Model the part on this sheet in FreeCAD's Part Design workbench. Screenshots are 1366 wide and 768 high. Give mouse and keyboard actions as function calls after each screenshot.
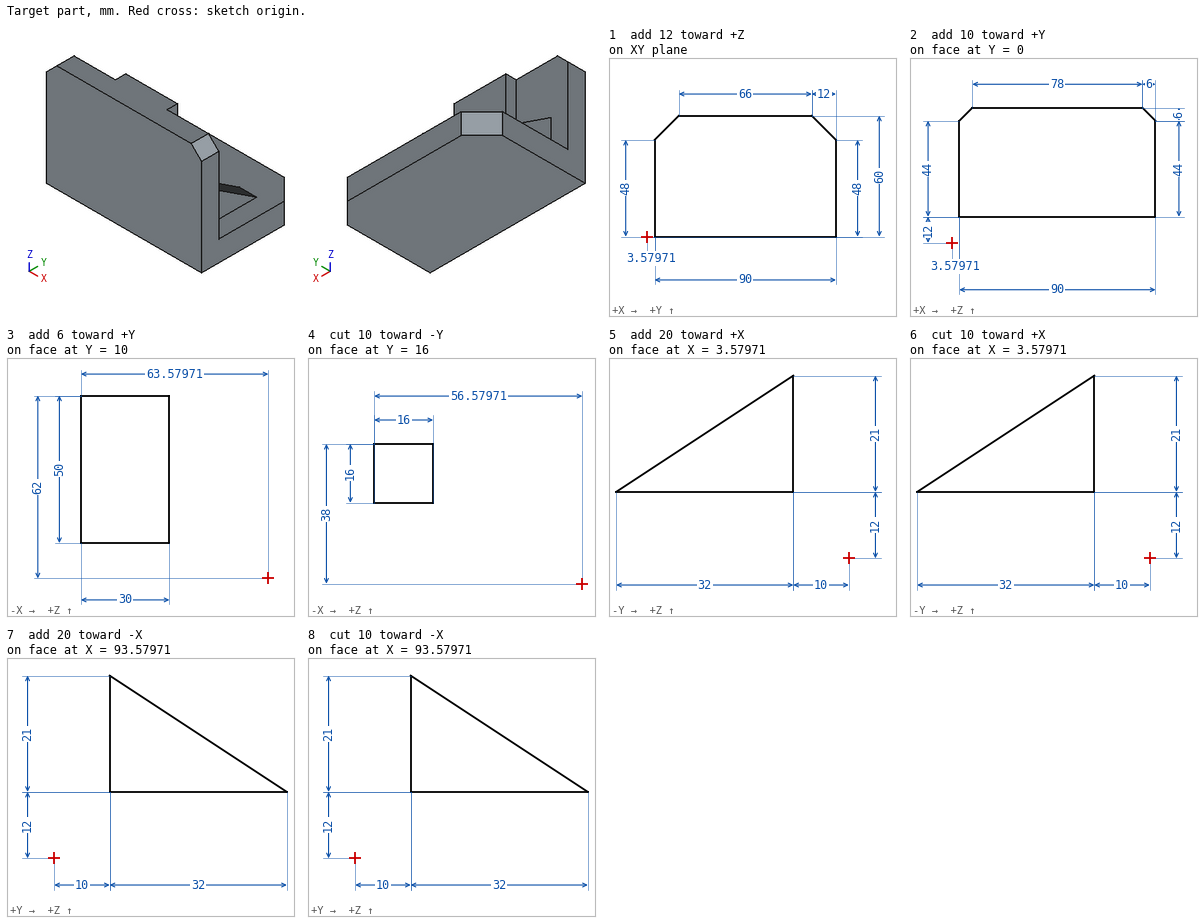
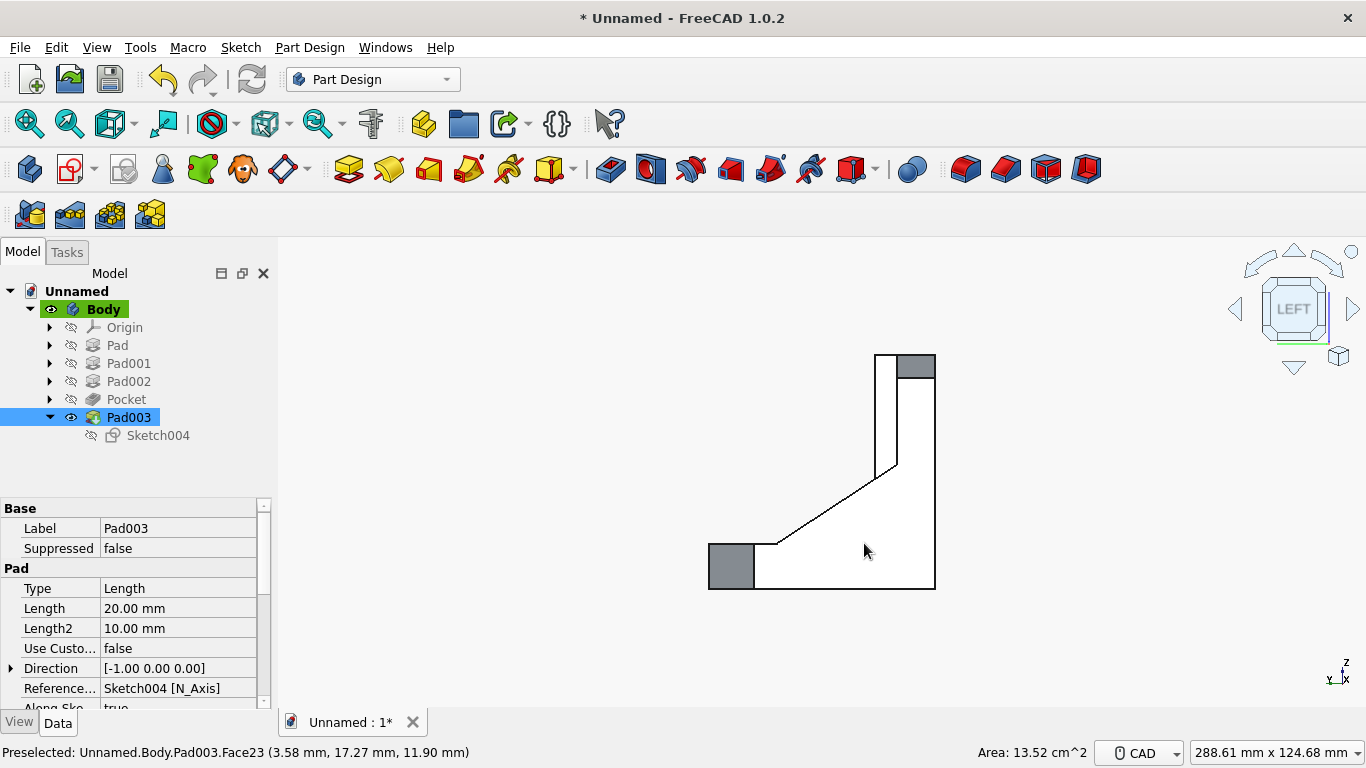
click(70, 170)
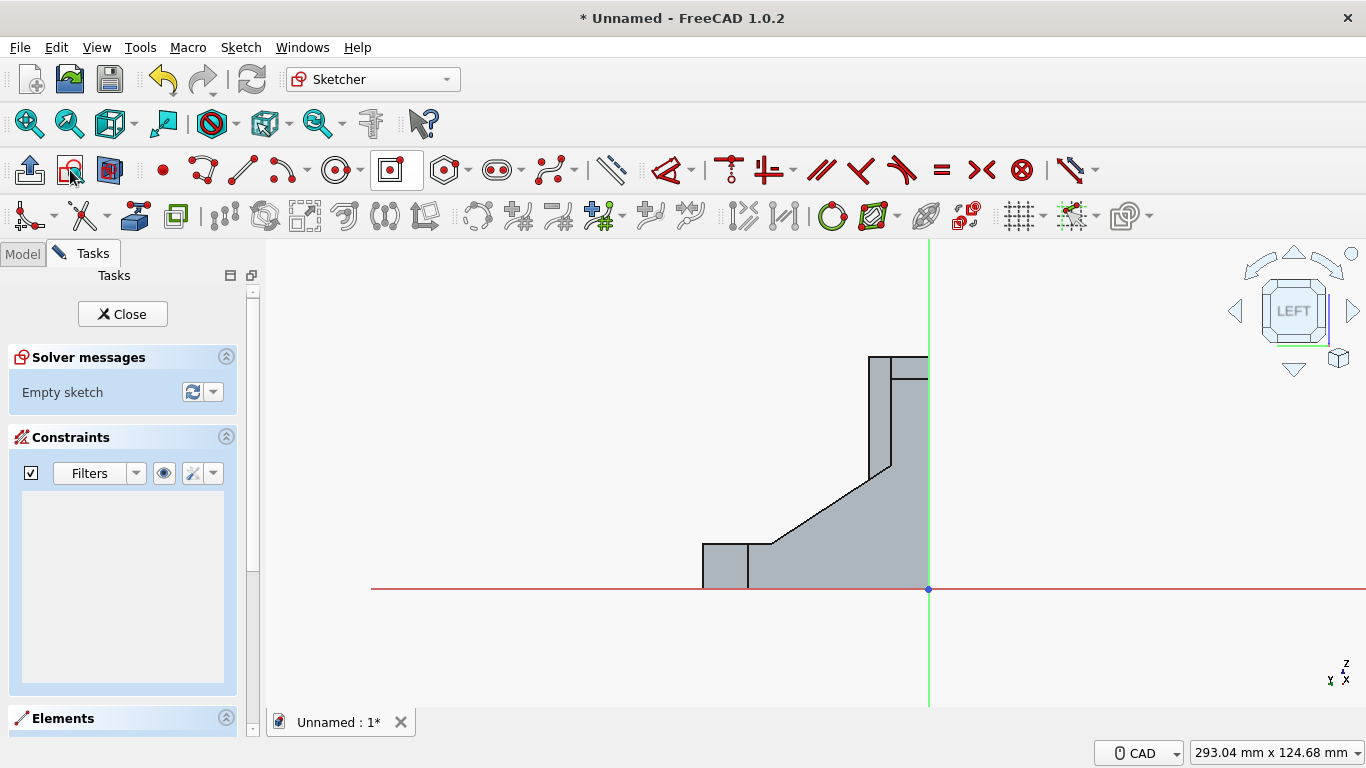
scroll(933, 572, up, 4)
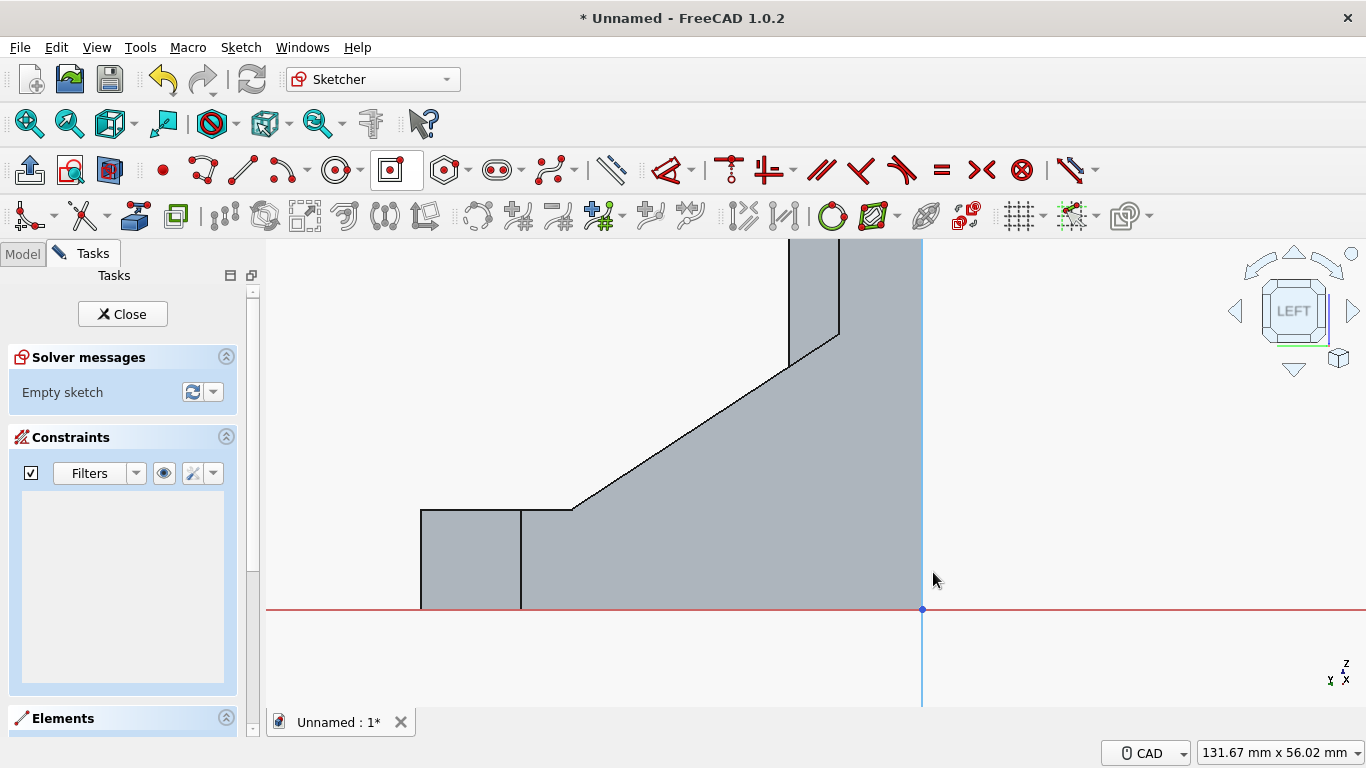
key(g)
key(m)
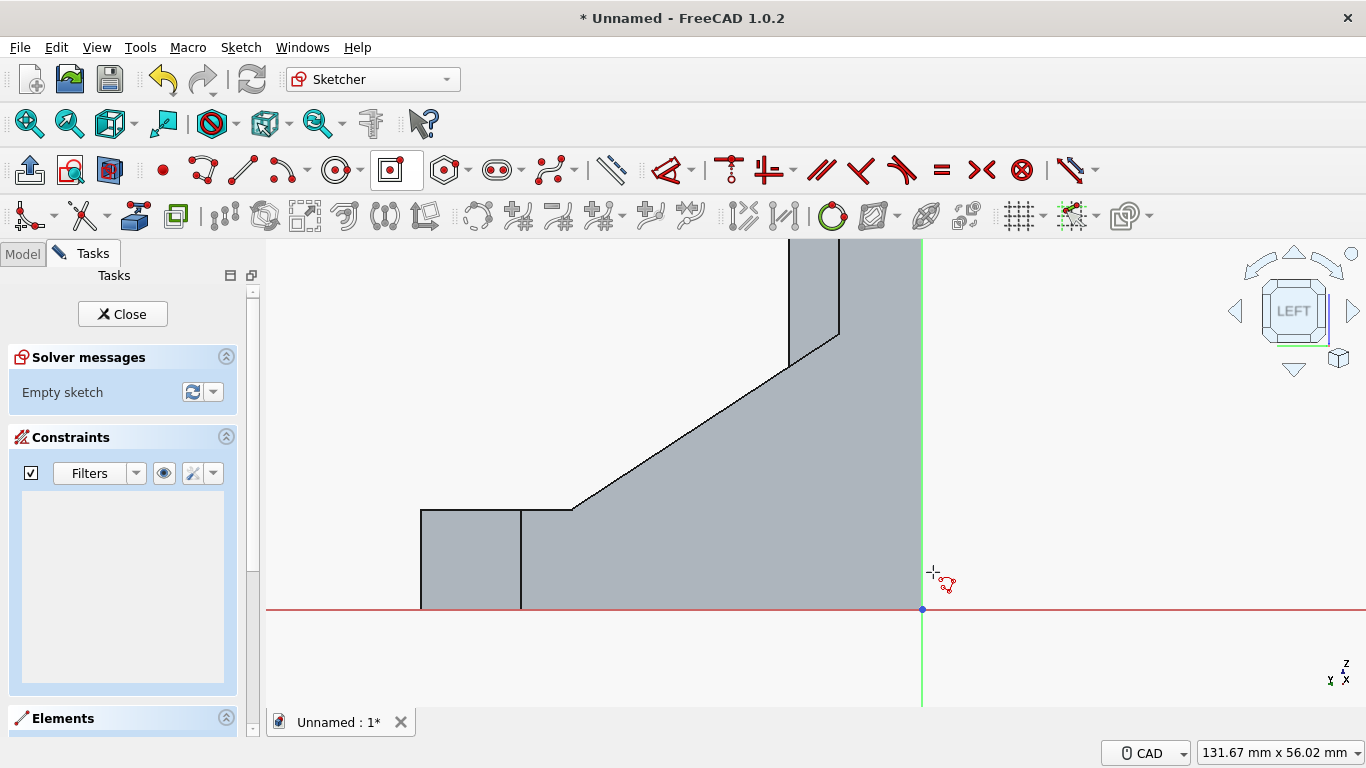
click(839, 510)
click(839, 334)
click(572, 510)
click(839, 511)
key(Escape)
key(Escape)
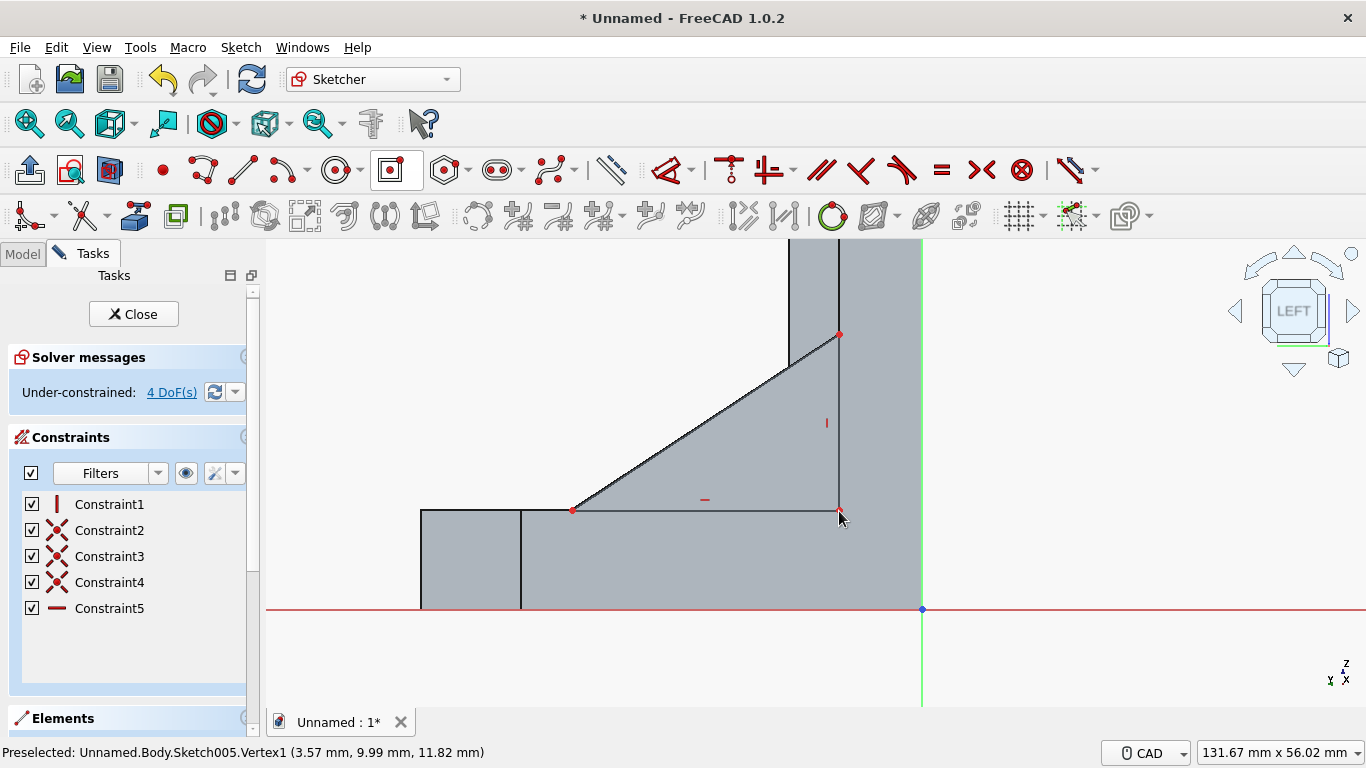
key(d)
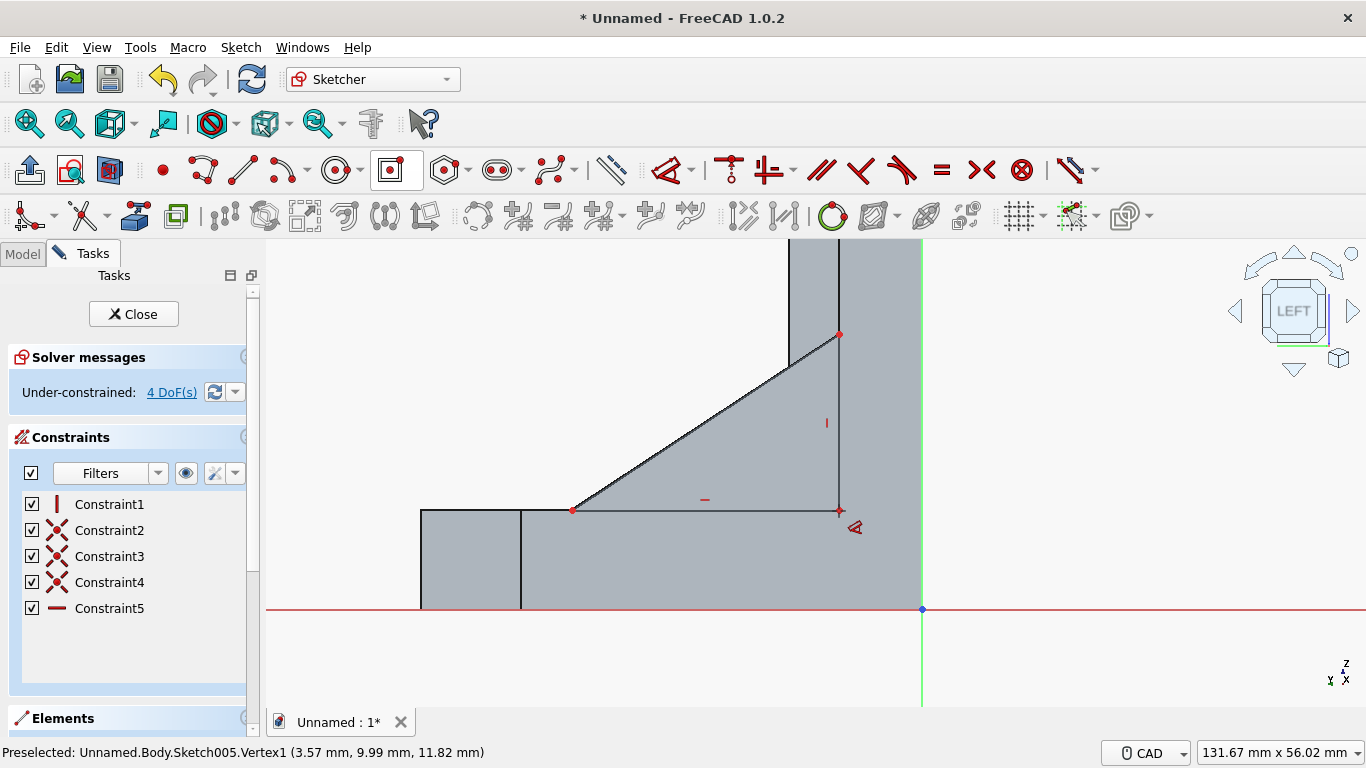
click(839, 458)
click(873, 423)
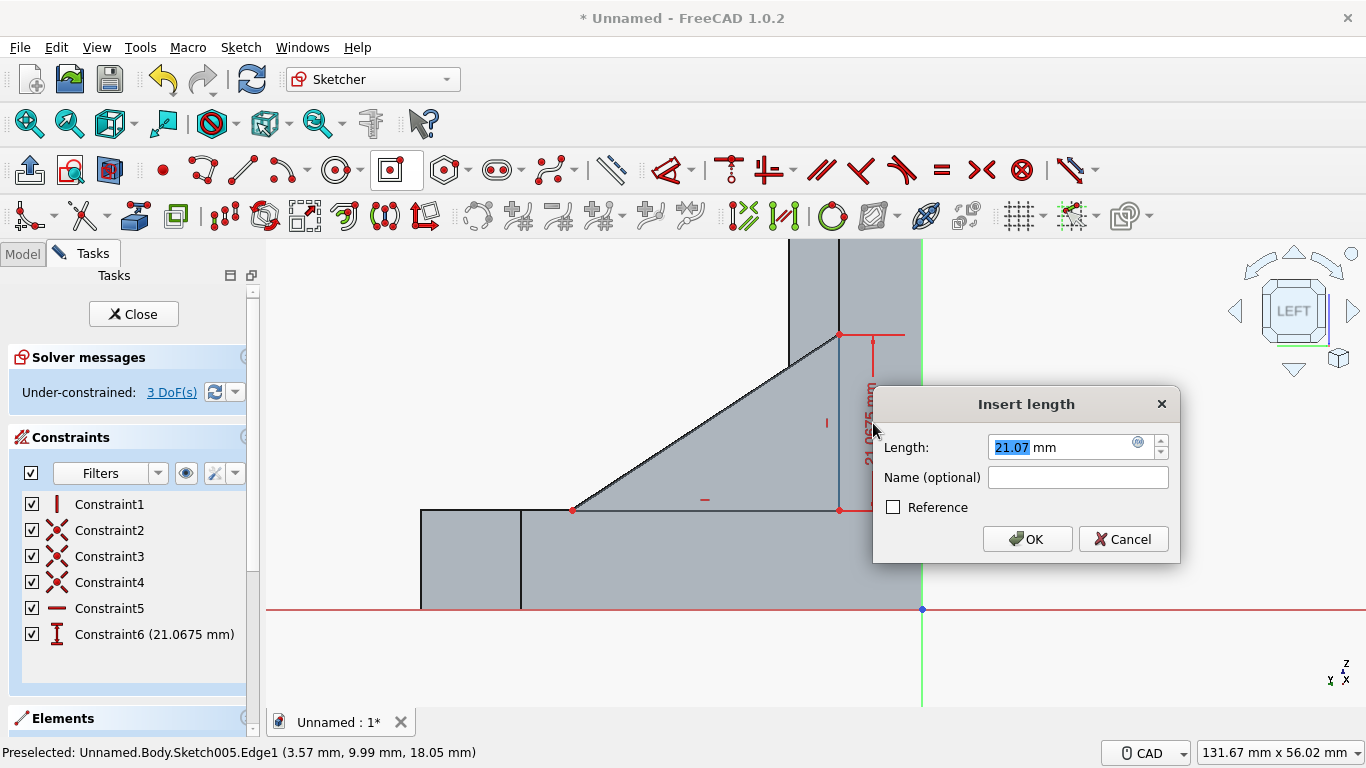
text(21)
key(Return)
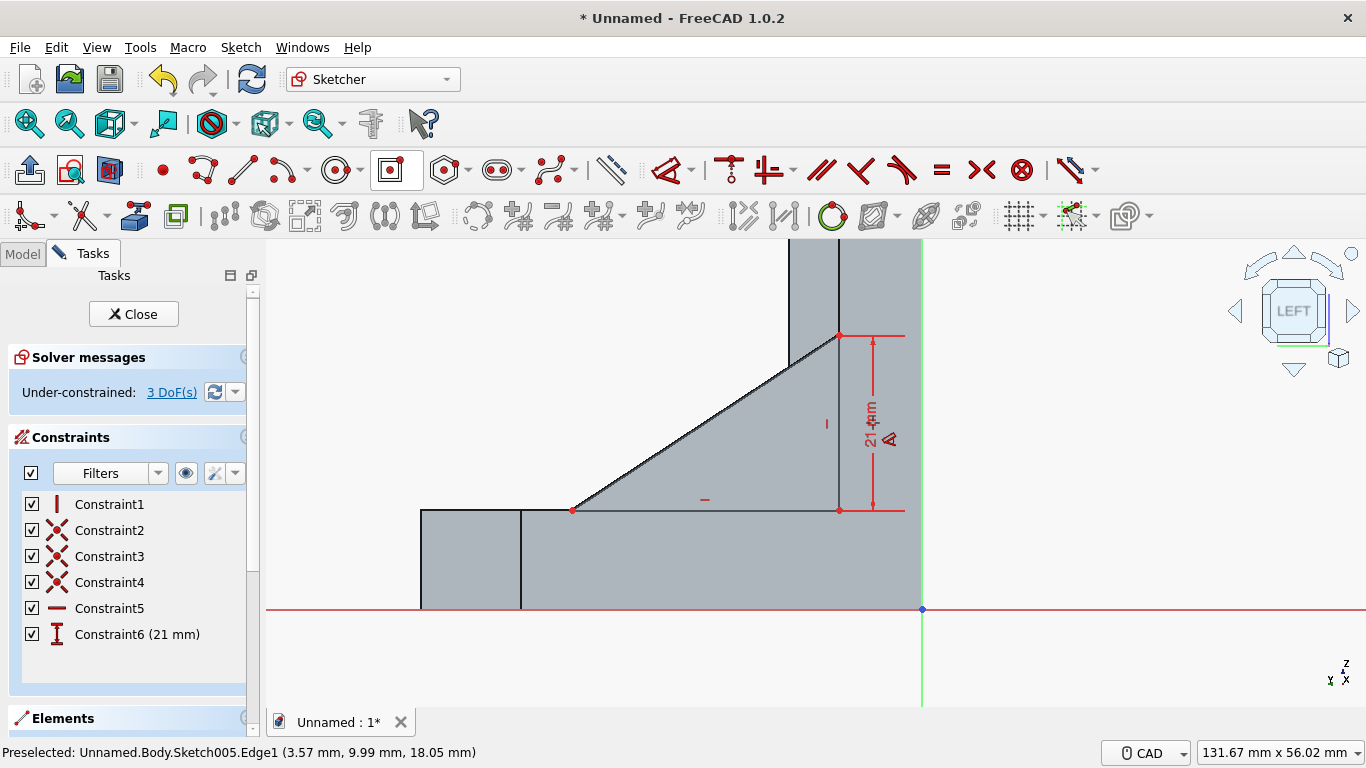
click(652, 511)
click(705, 545)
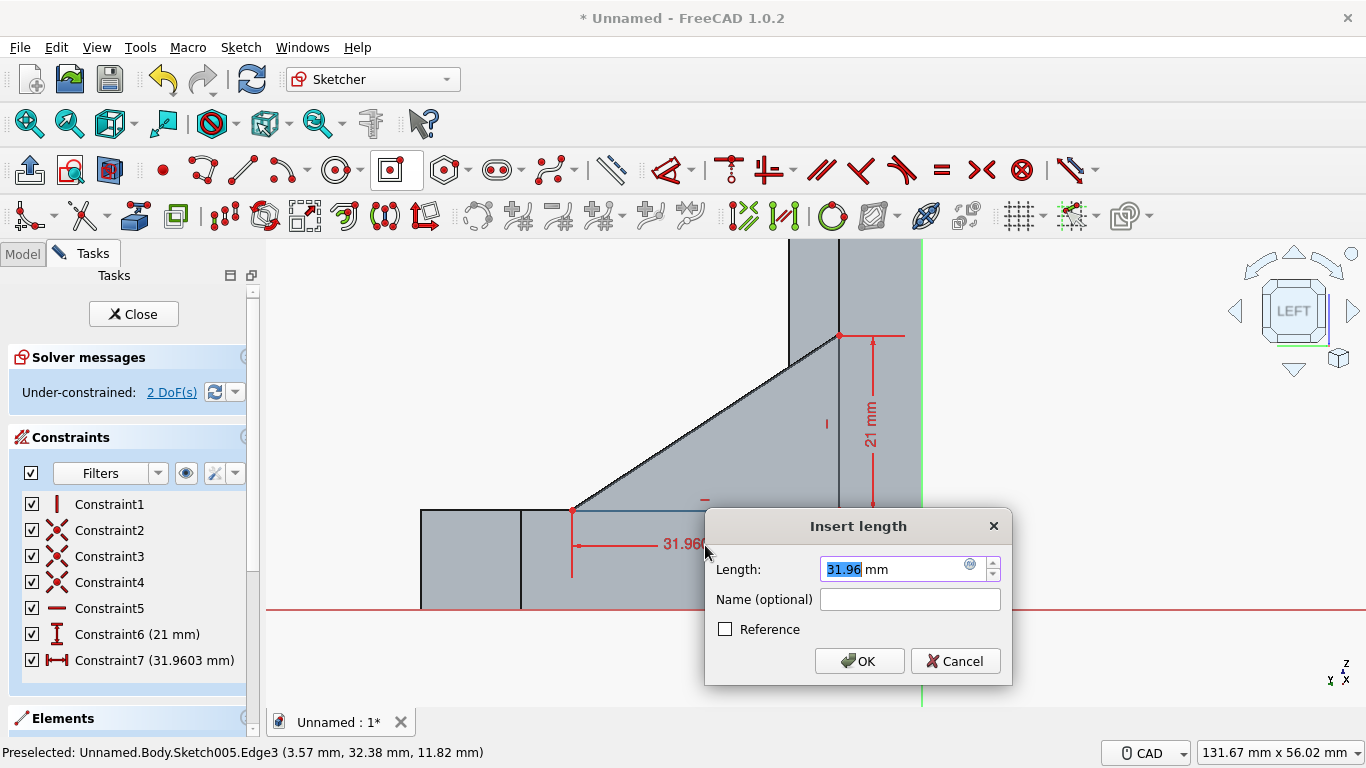
text(32)
key(Return)